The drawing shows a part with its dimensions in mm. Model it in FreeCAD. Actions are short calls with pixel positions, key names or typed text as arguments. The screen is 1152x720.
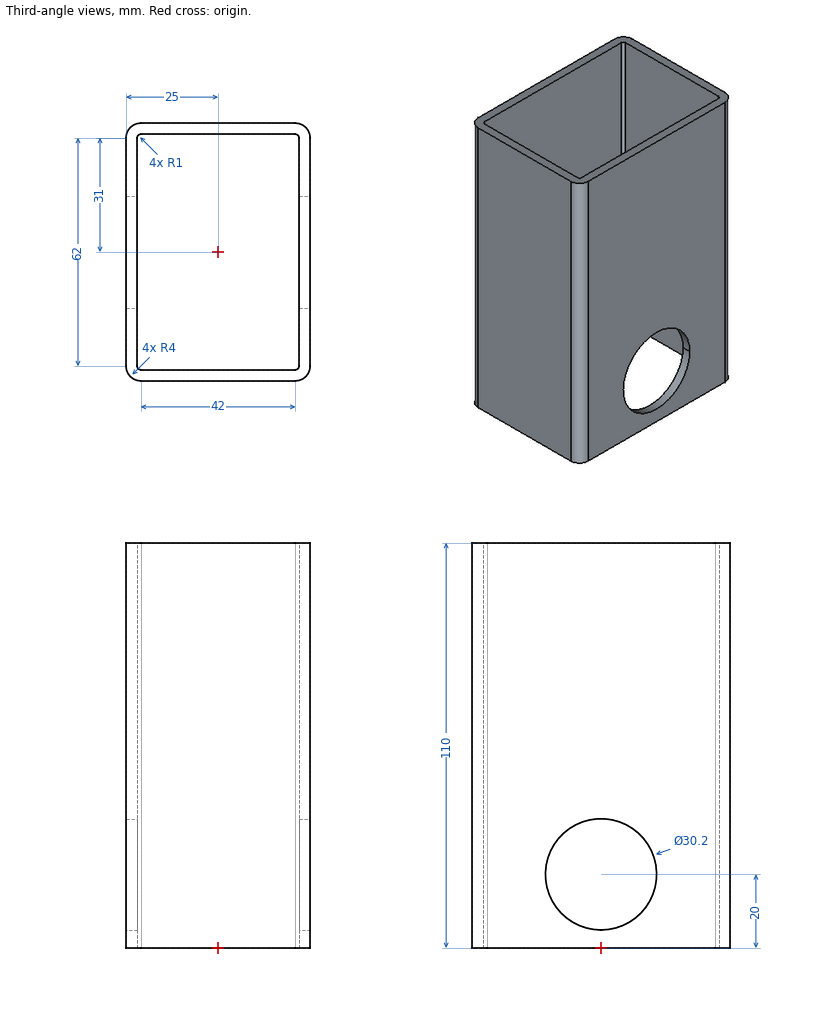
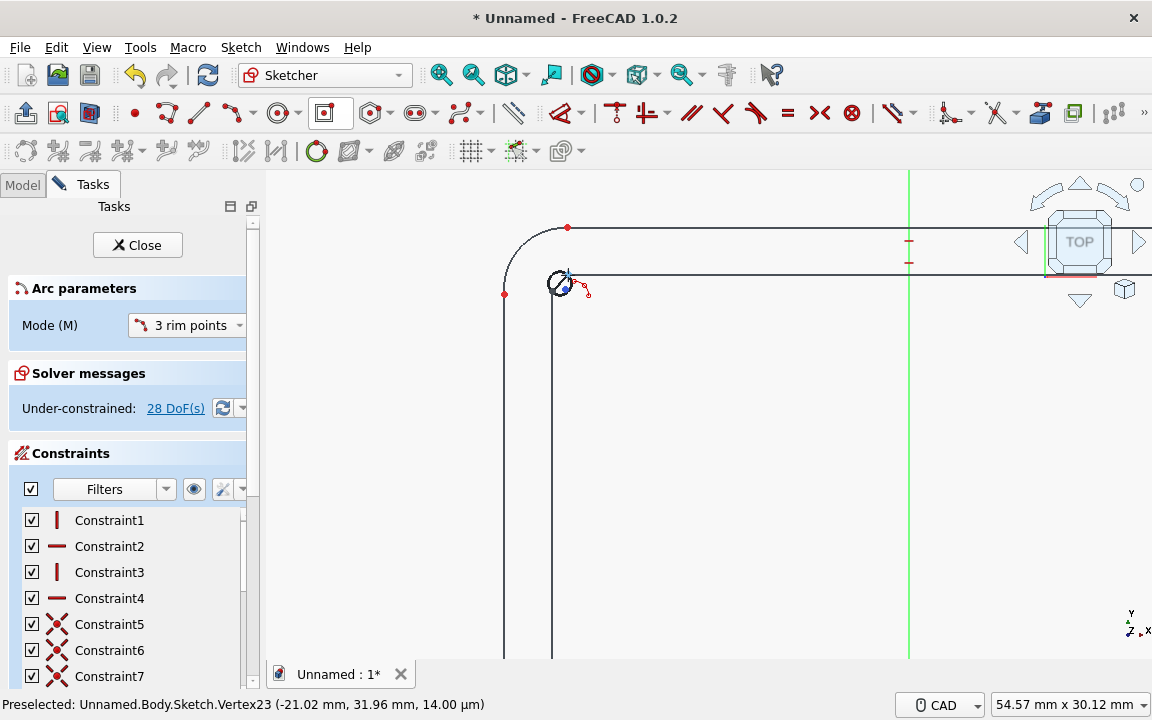
scroll(557, 279, up, 7)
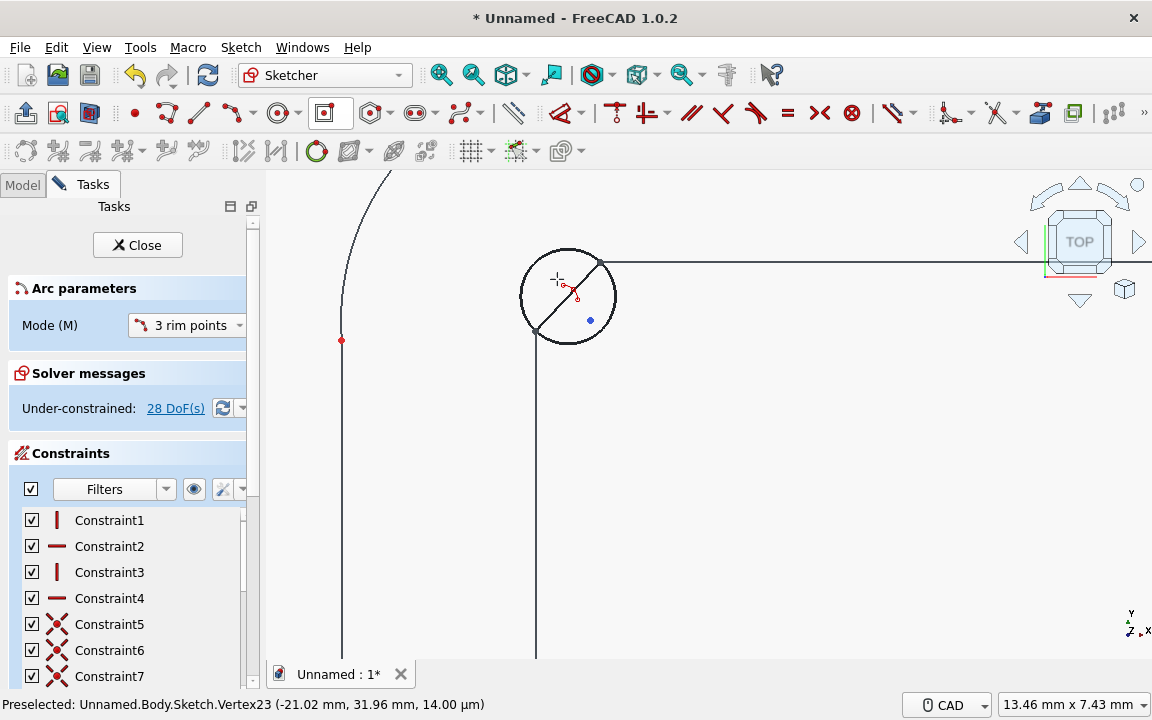
click(555, 279)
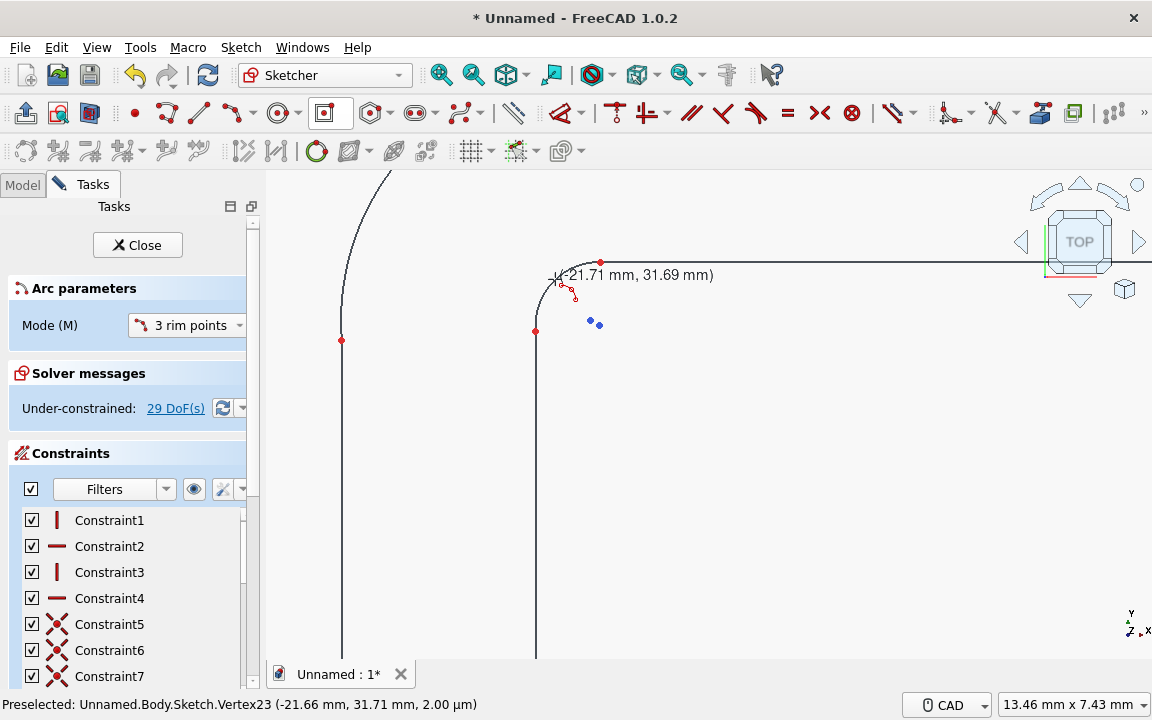
scroll(553, 288, down, 14)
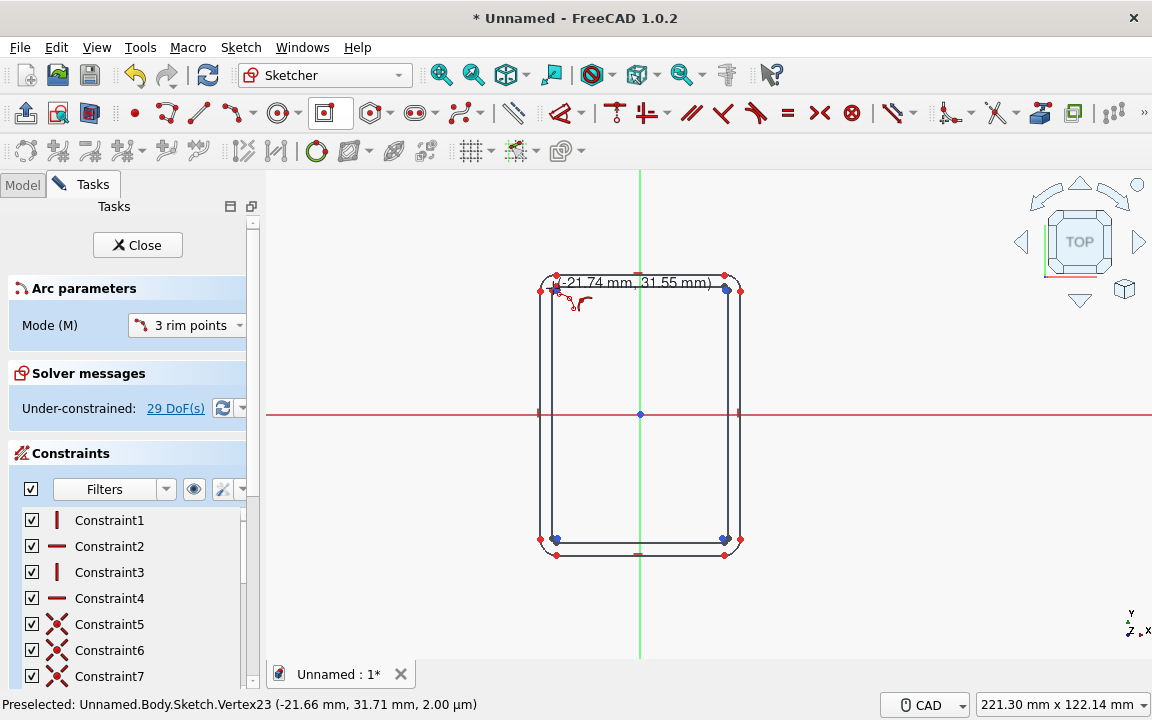
scroll(724, 287, up, 7)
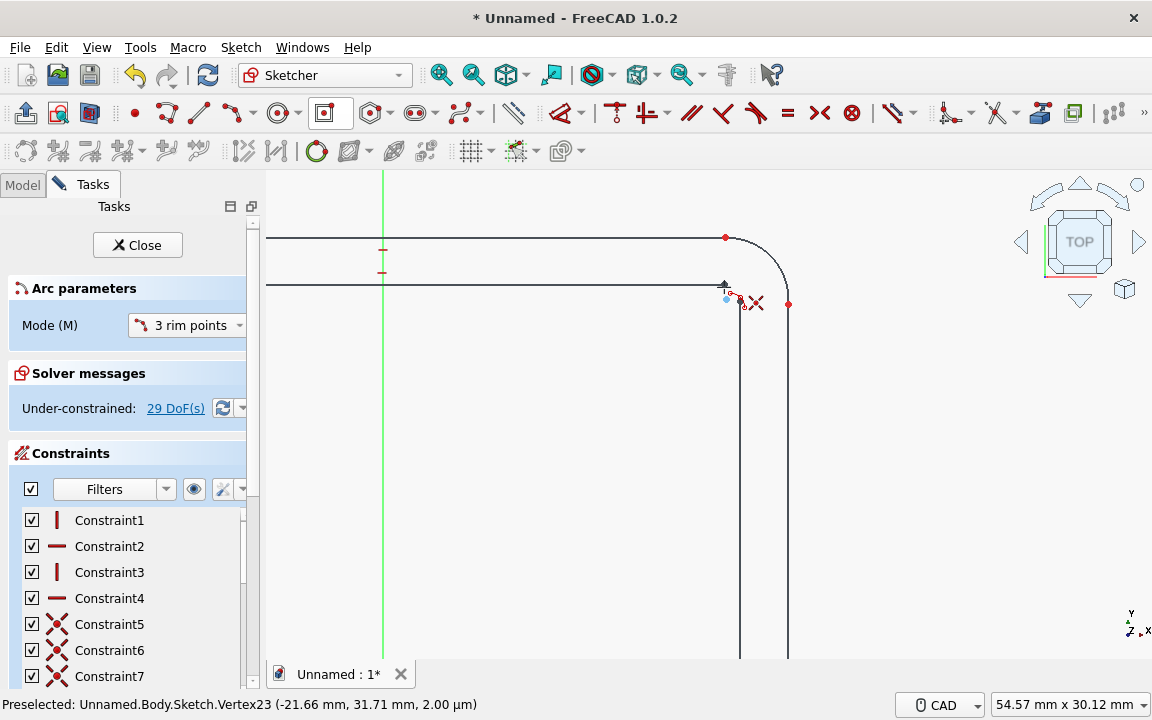
click(724, 285)
click(740, 302)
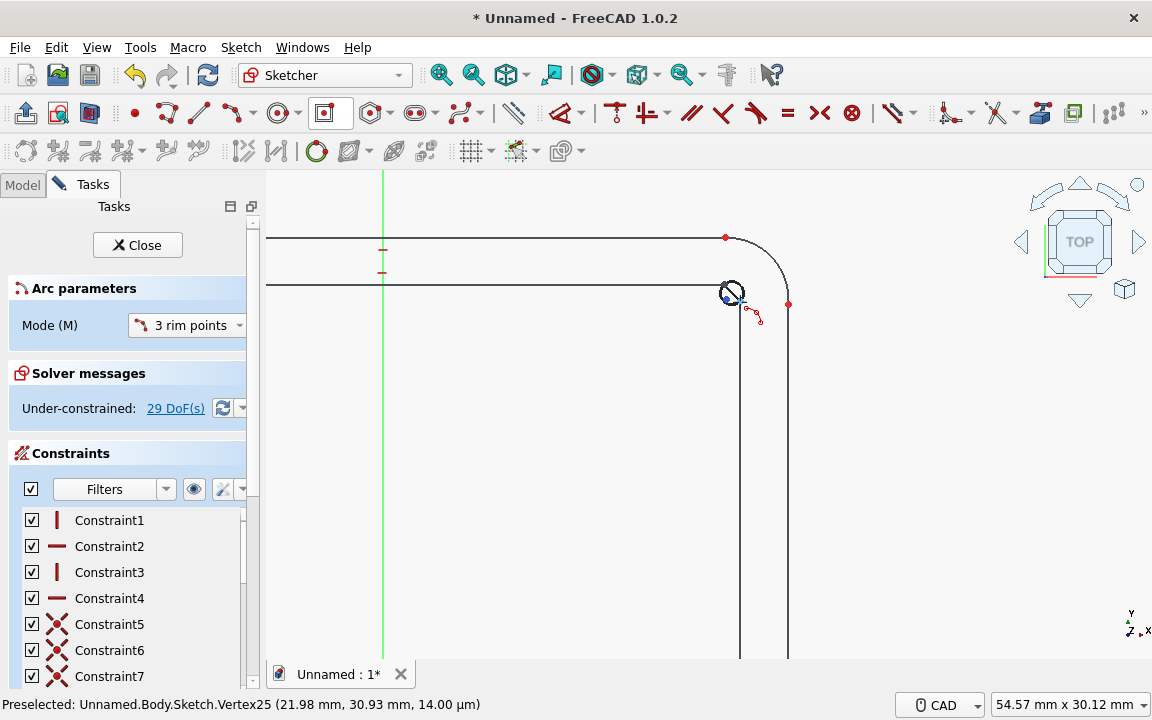
scroll(736, 289, up, 7)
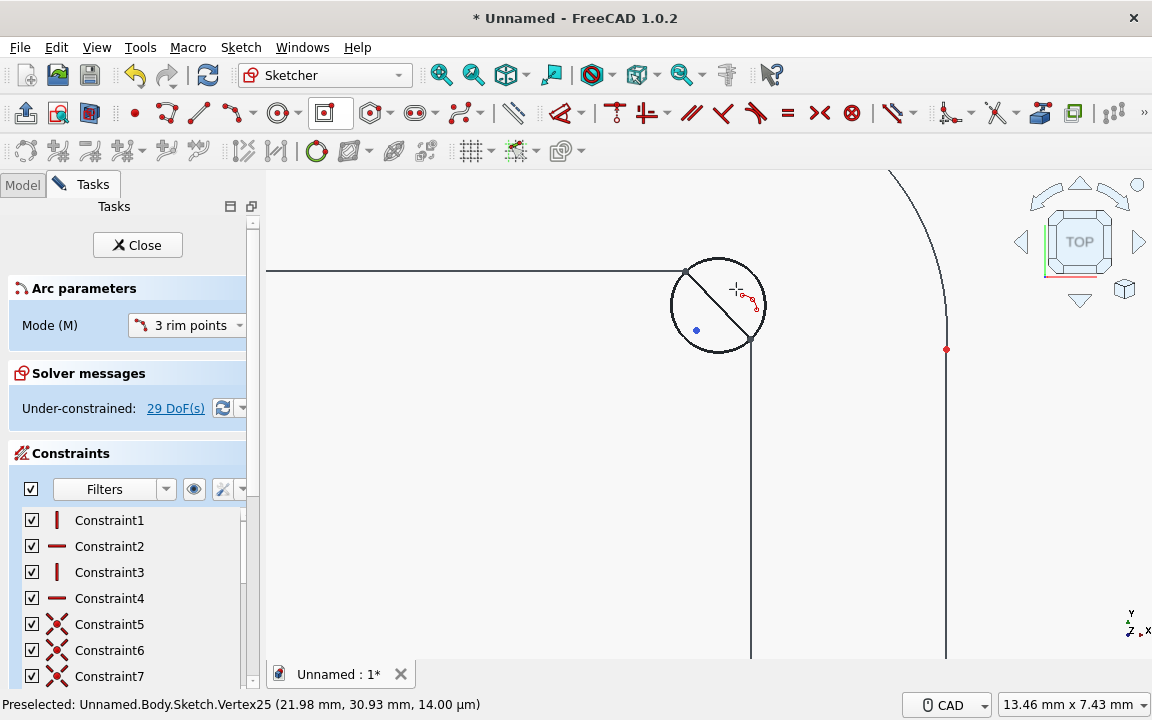
click(733, 288)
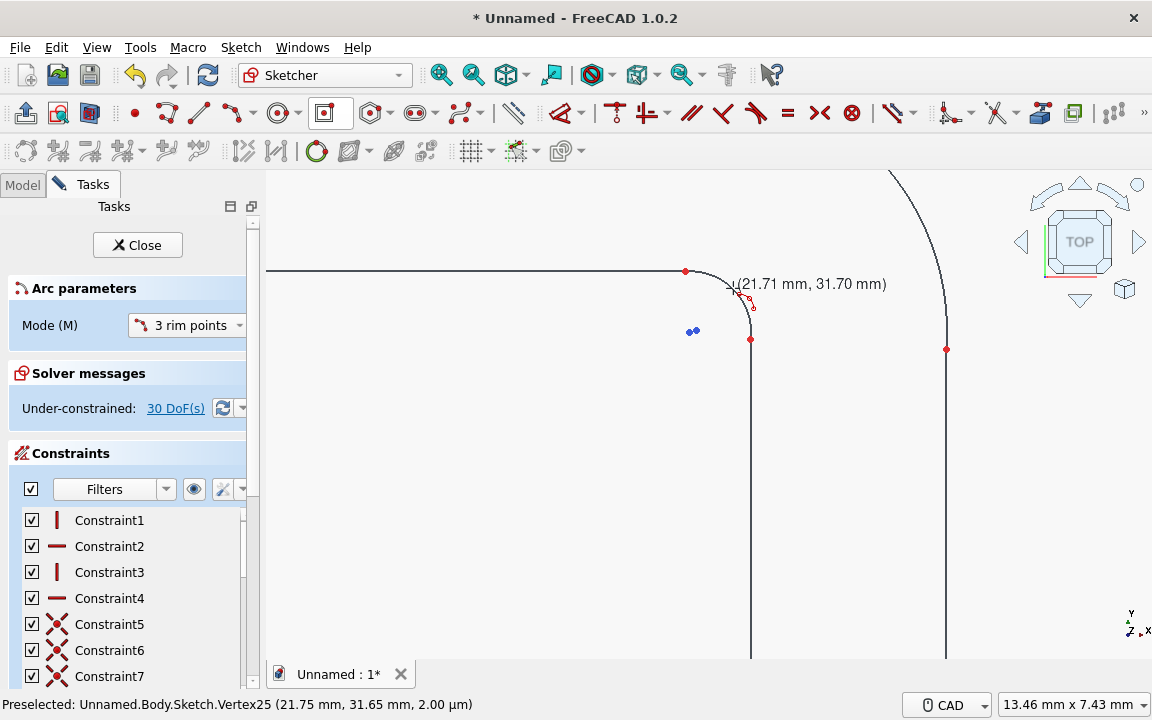
scroll(727, 288, down, 14)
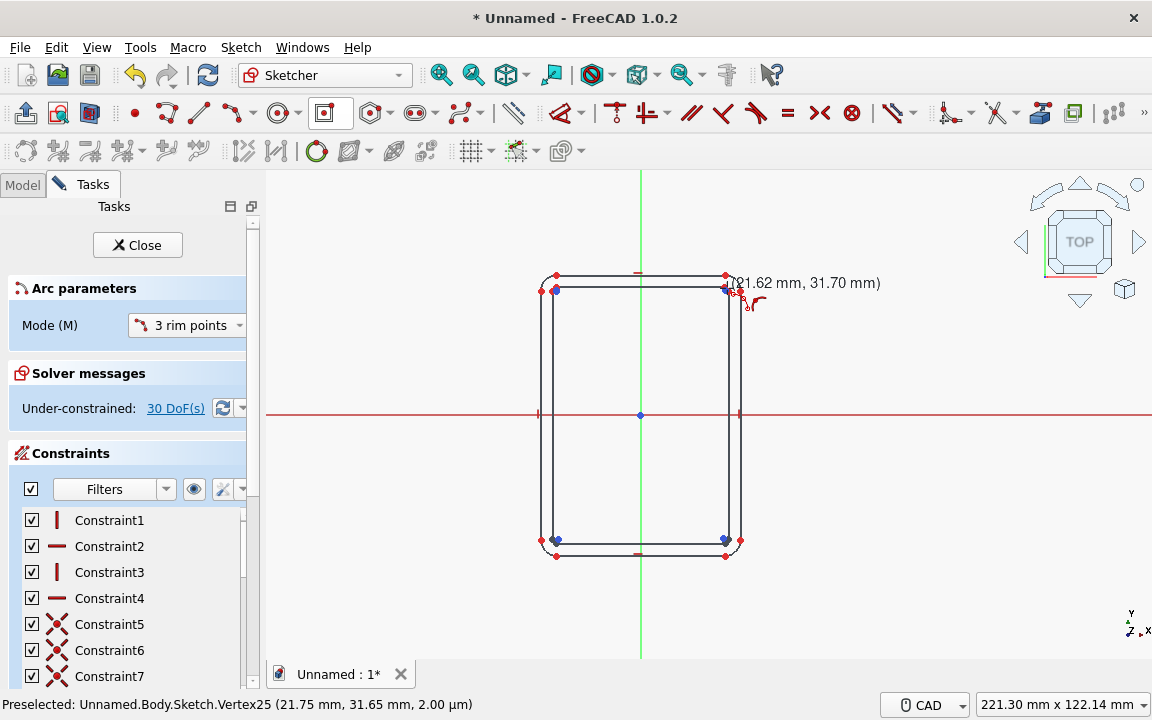
scroll(729, 539, up, 7)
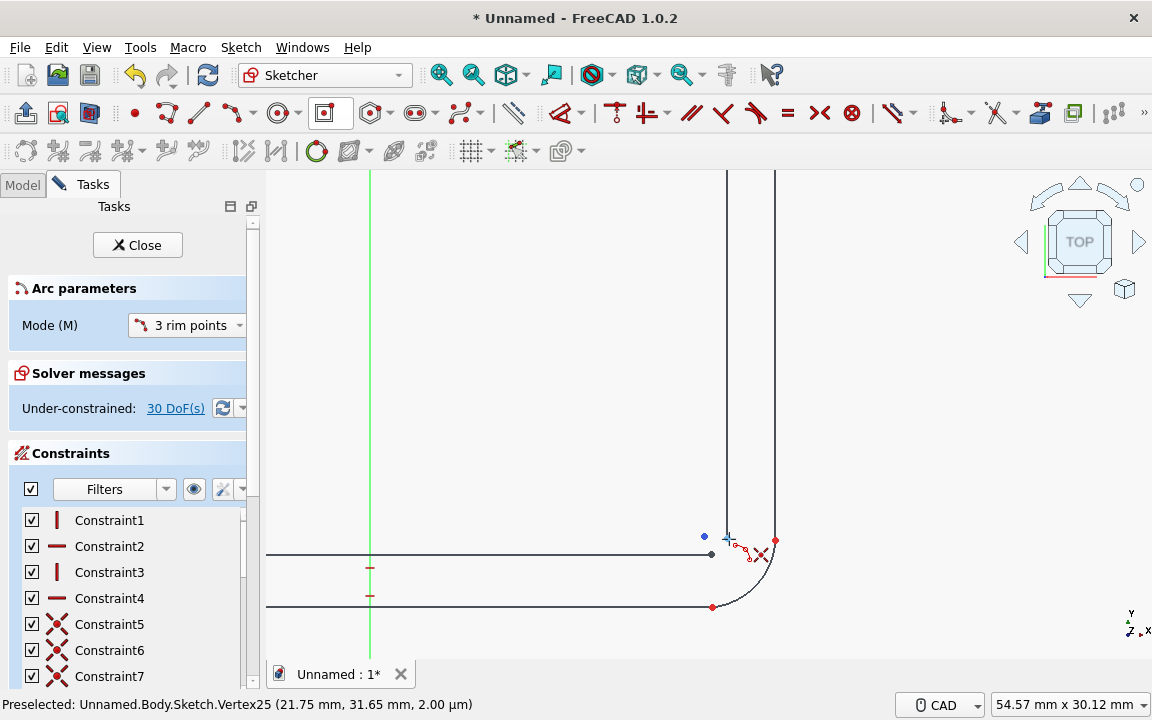
click(727, 539)
click(711, 555)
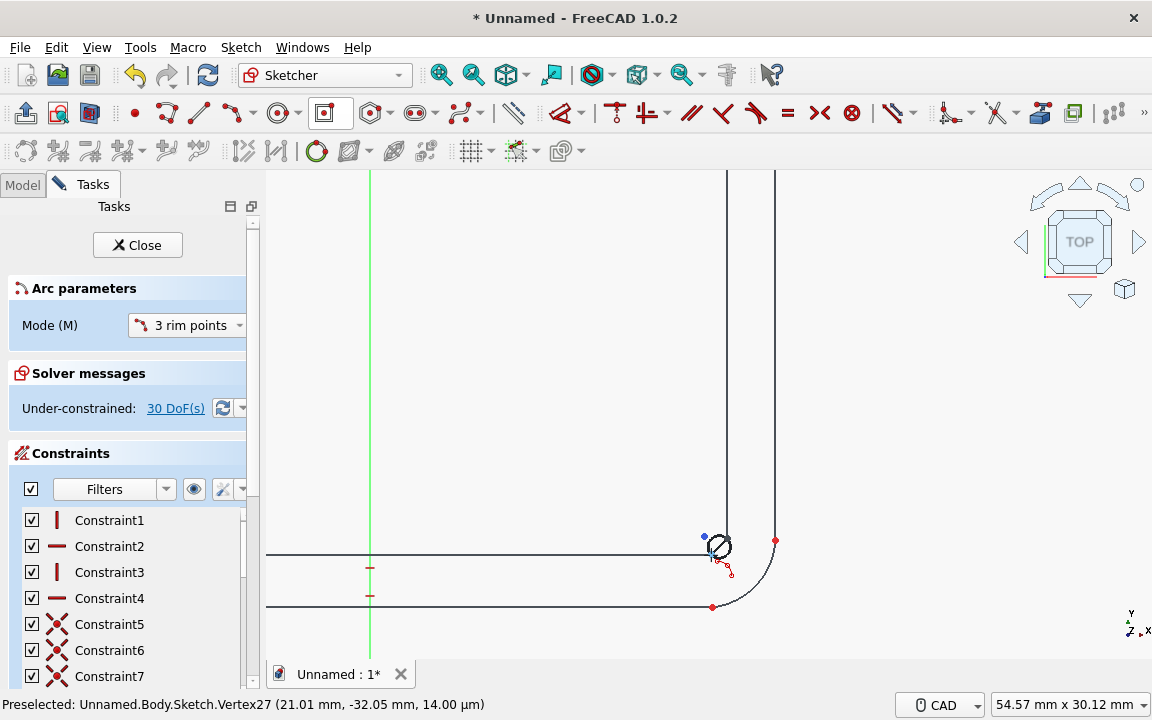
scroll(723, 549, up, 7)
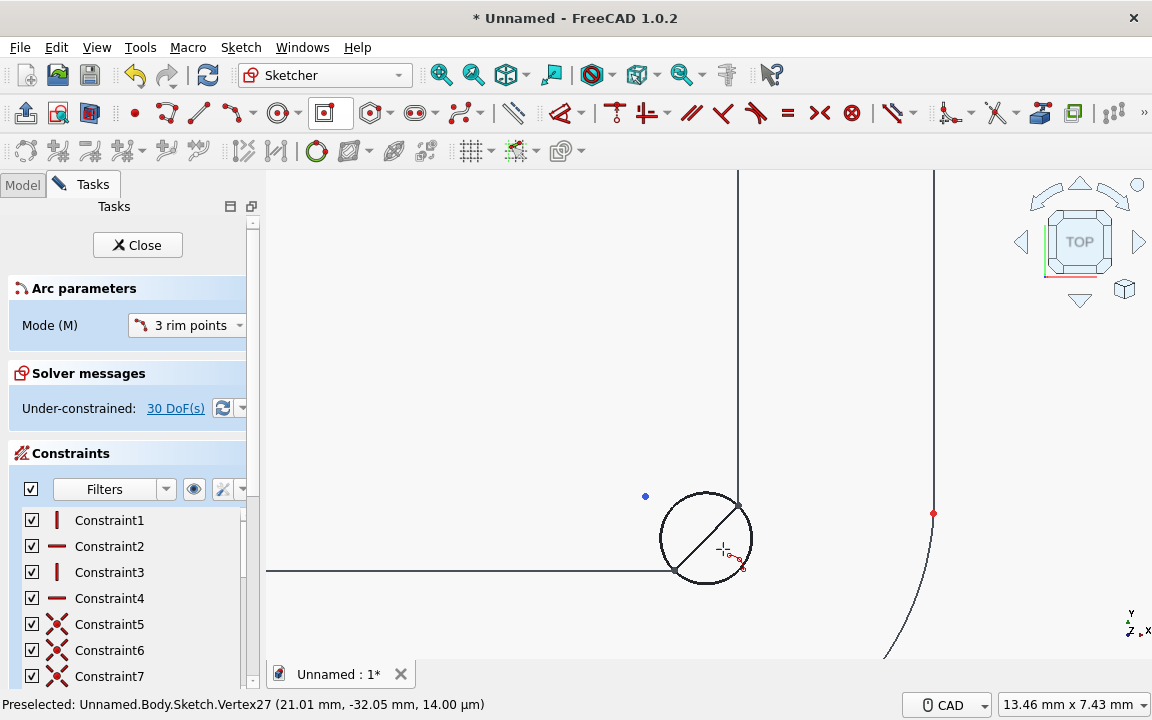
click(720, 548)